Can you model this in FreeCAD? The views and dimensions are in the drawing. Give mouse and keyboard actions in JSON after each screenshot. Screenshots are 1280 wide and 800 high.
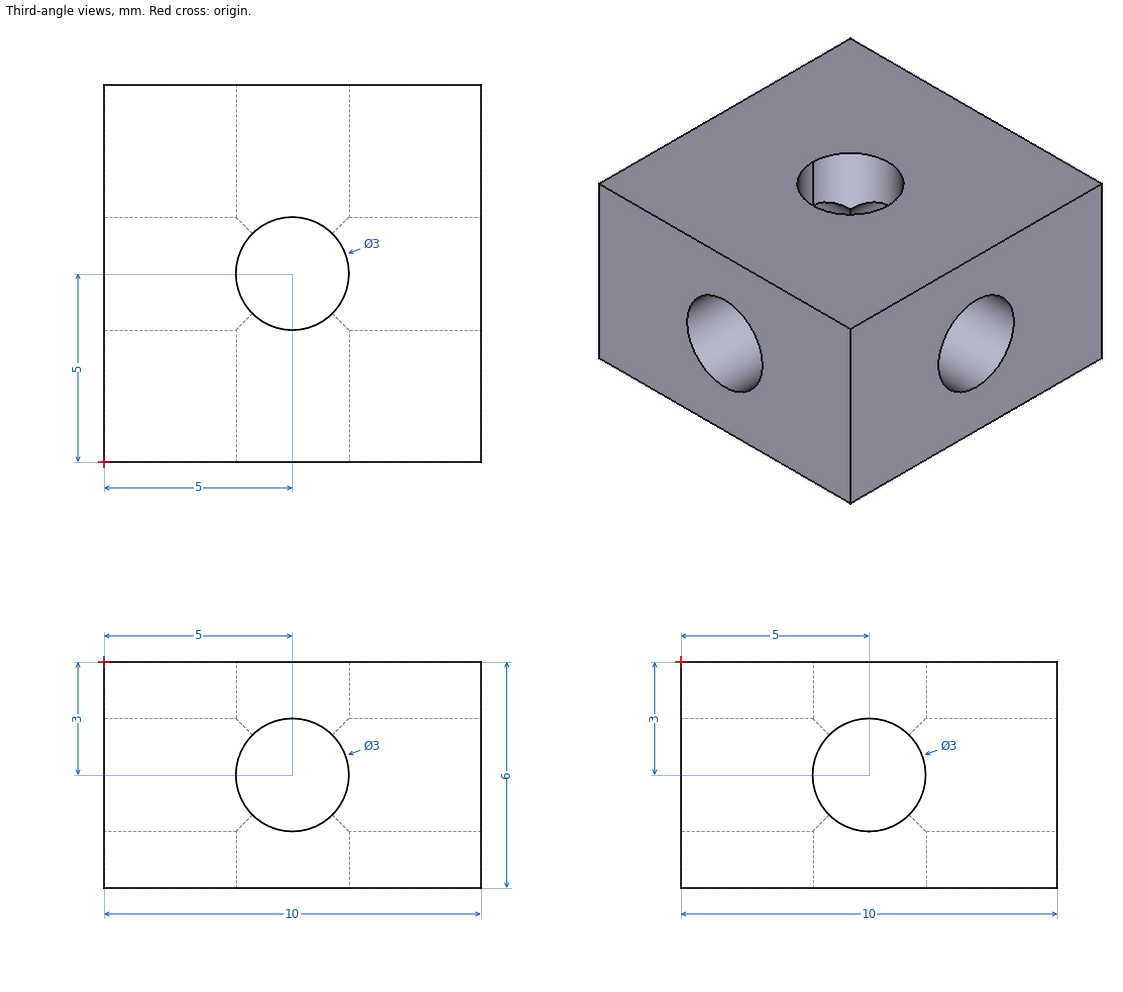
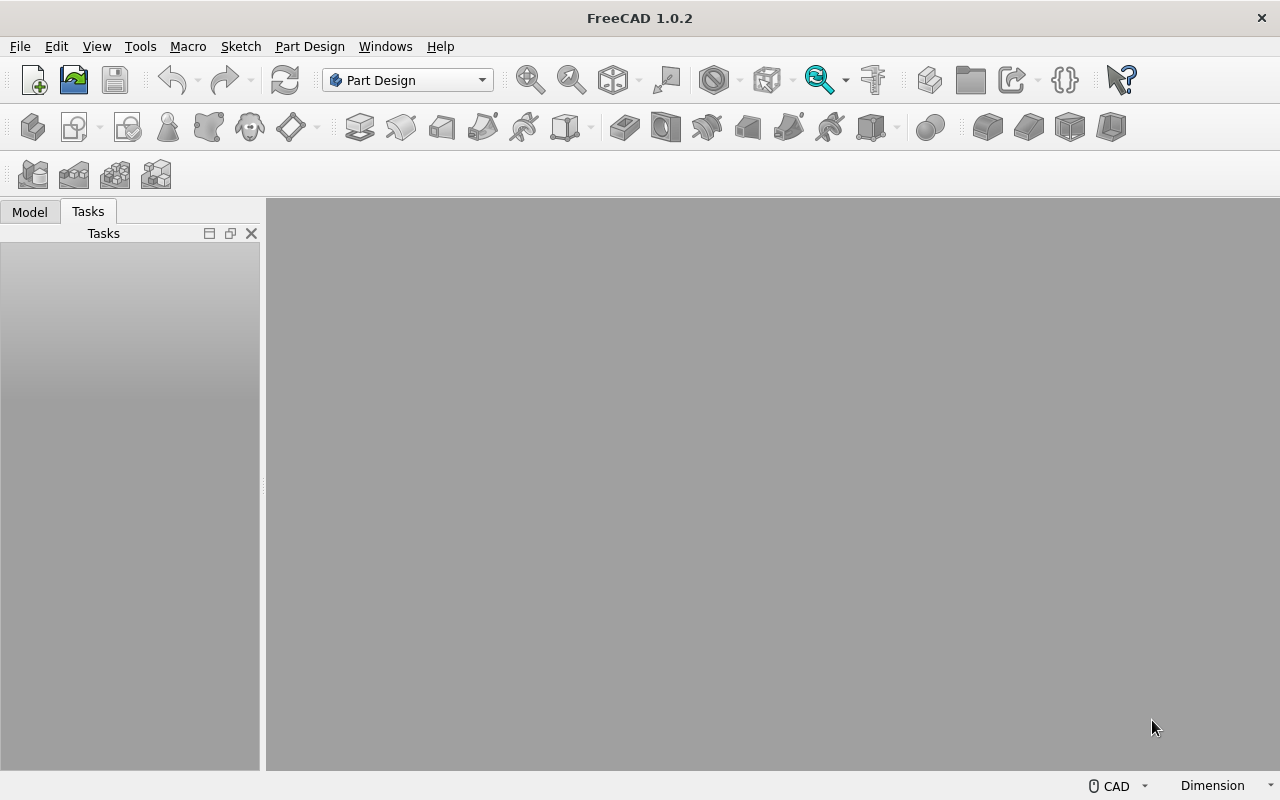
{"action": "left_click", "coordinate": [33, 80]}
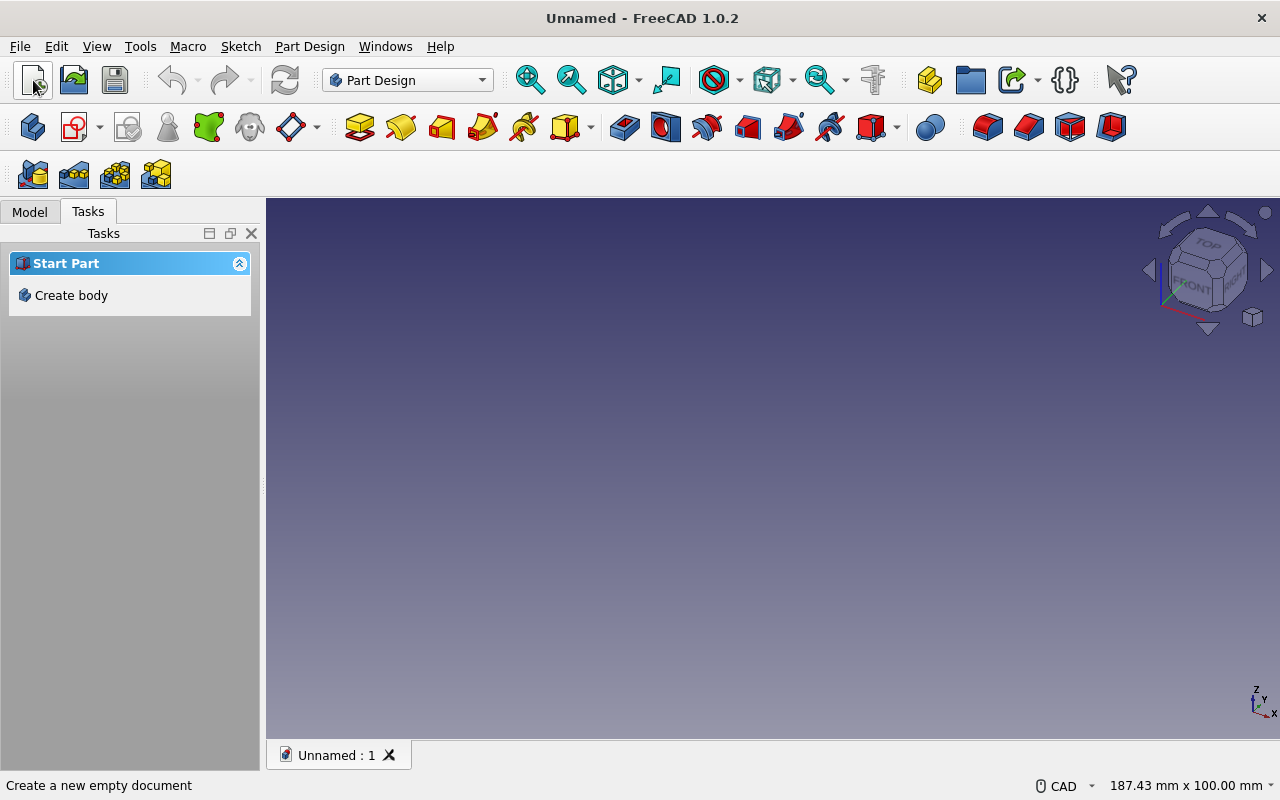
{"action": "left_click", "coordinate": [74, 128]}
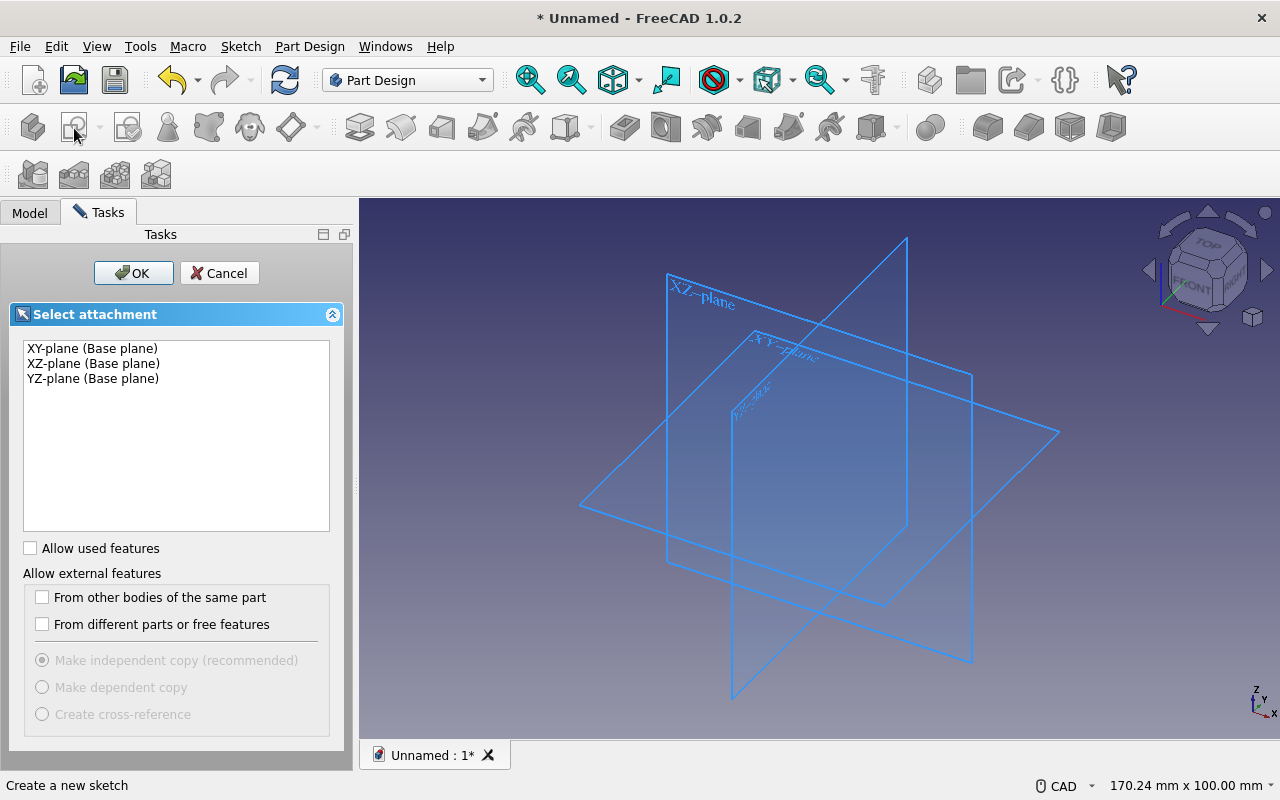
{"action": "left_click", "coordinate": [84, 364]}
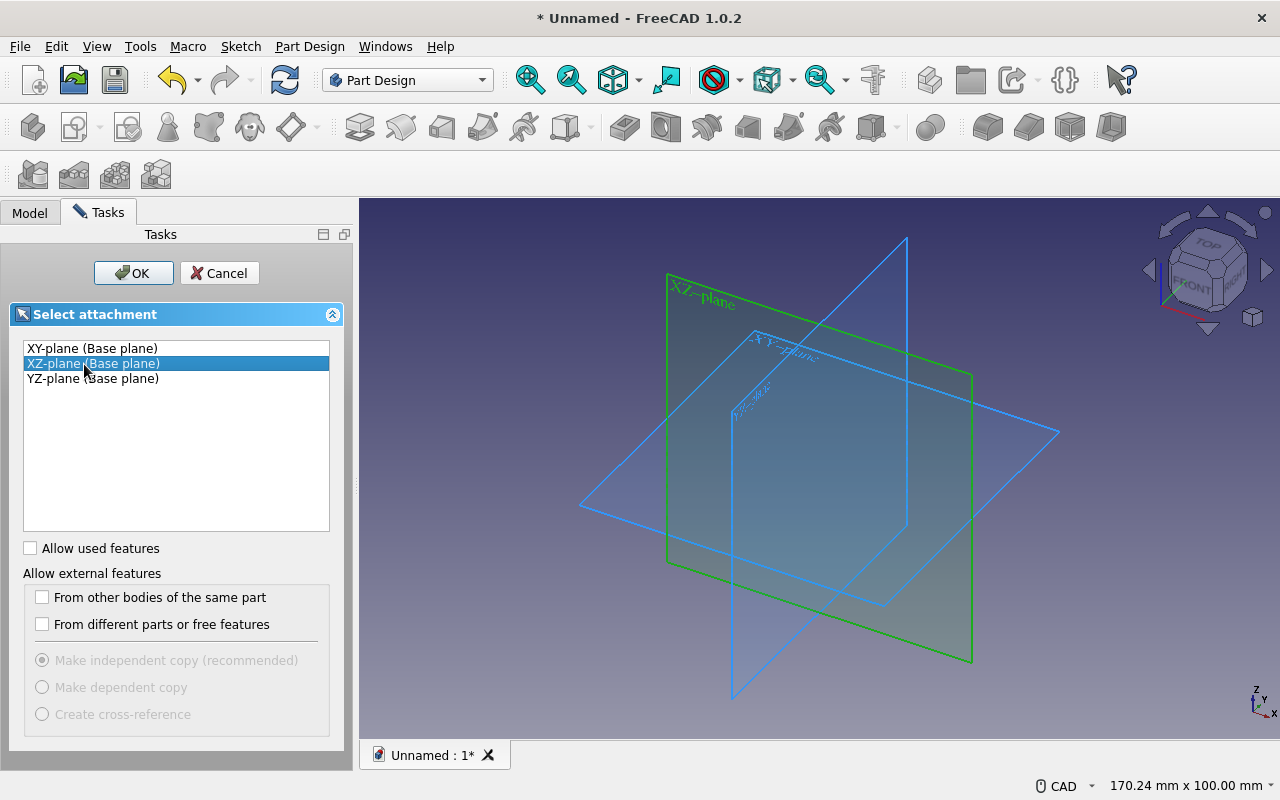
{"action": "left_click", "coordinate": [134, 273]}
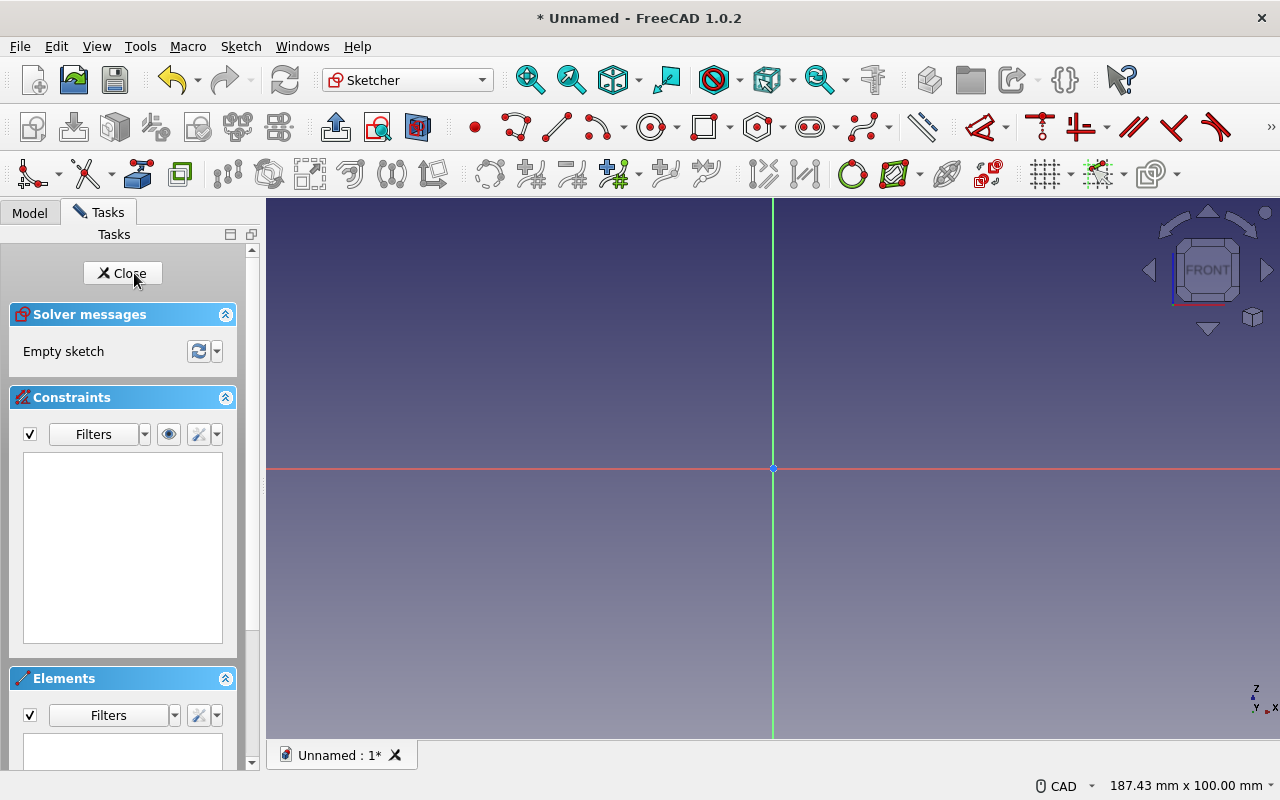
{"action": "scroll", "coordinate": [810, 486], "scroll_direction": "up", "scroll_amount": 12}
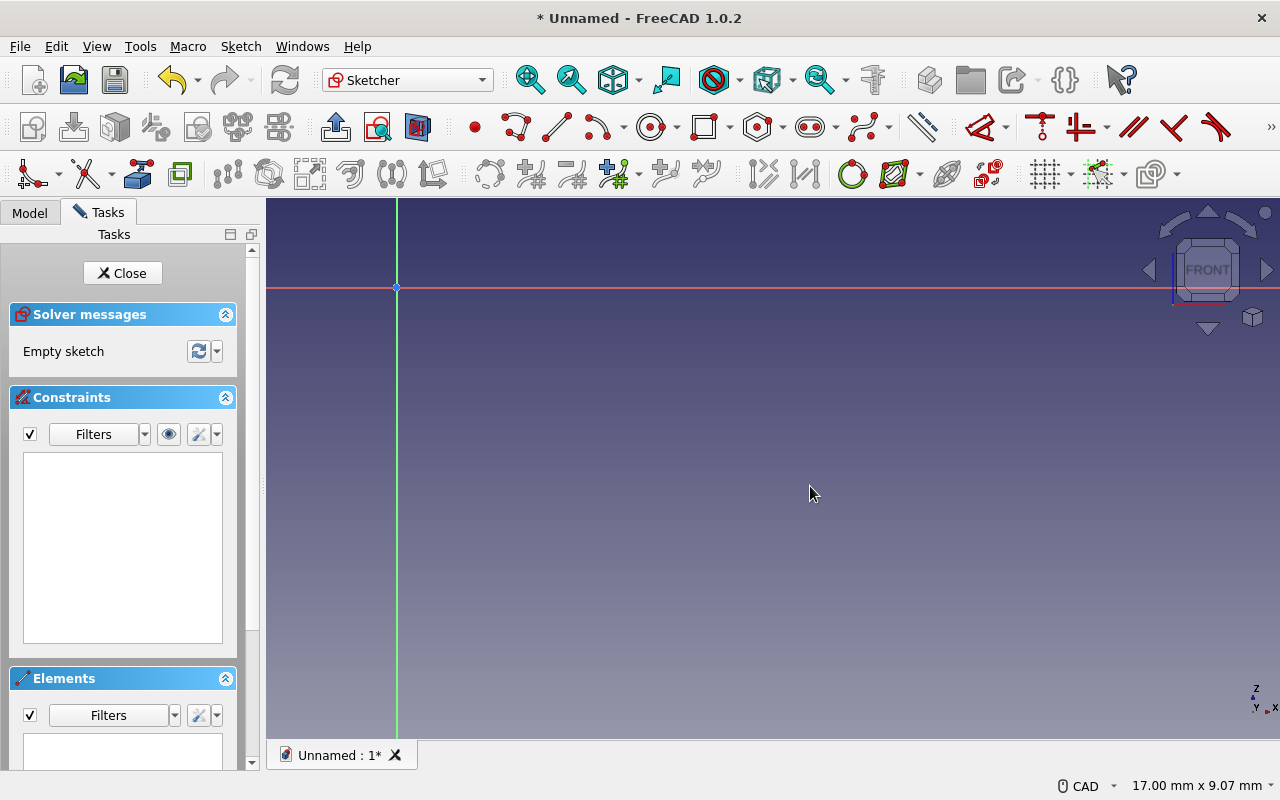
{"action": "left_click", "coordinate": [704, 128]}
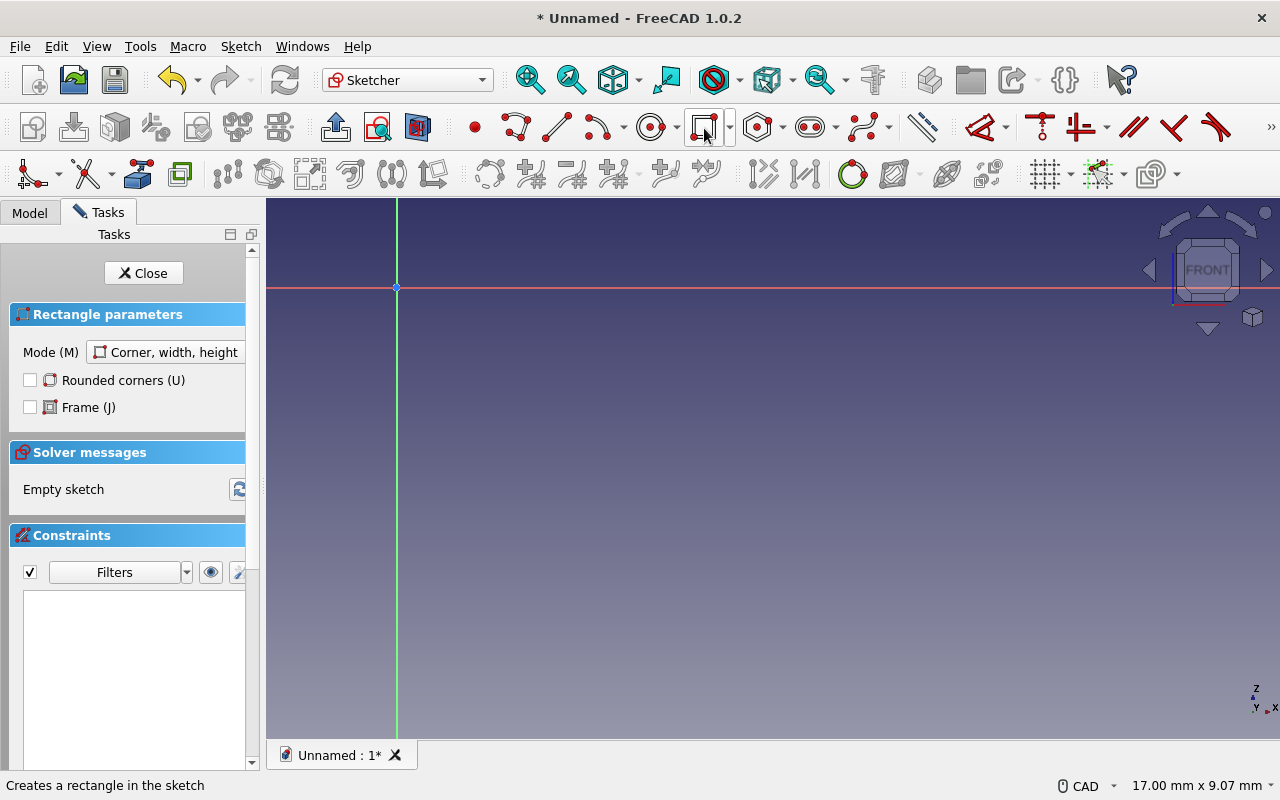
{"action": "left_click", "coordinate": [397, 288]}
{"action": "mouse_move", "coordinate": [993, 646]}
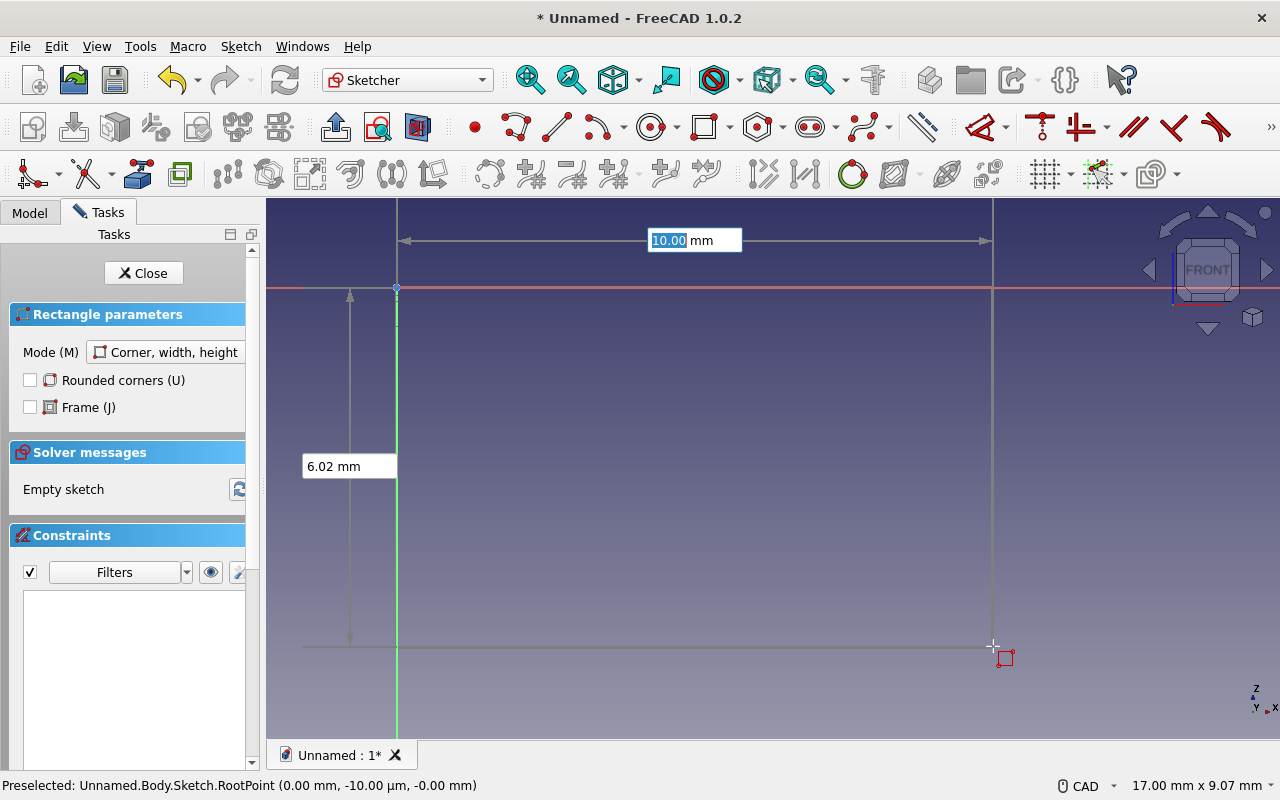
{"action": "type", "text": "10"}
{"action": "key", "text": "Tab"}
{"action": "type", "text": "6"}
{"action": "key", "text": "Return"}
{"action": "key", "text": "Escape"}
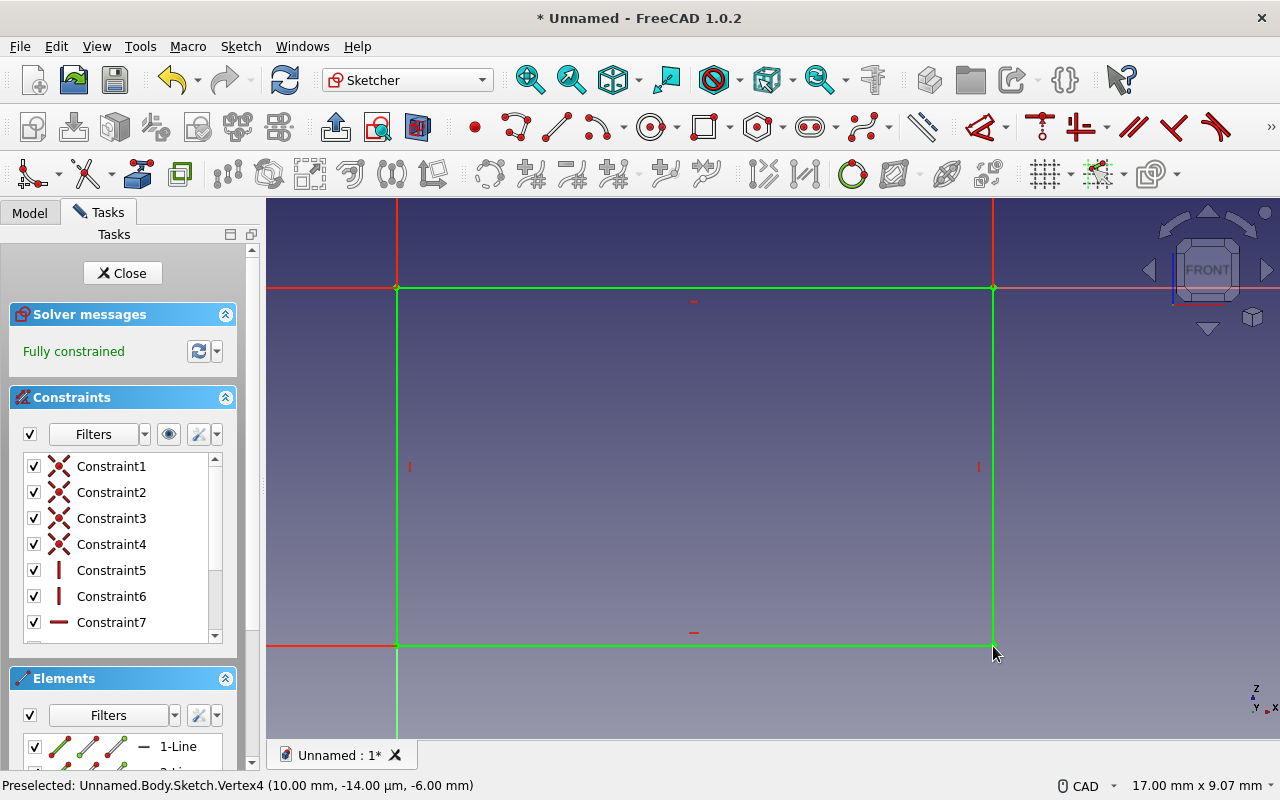
{"action": "left_click", "coordinate": [123, 273]}